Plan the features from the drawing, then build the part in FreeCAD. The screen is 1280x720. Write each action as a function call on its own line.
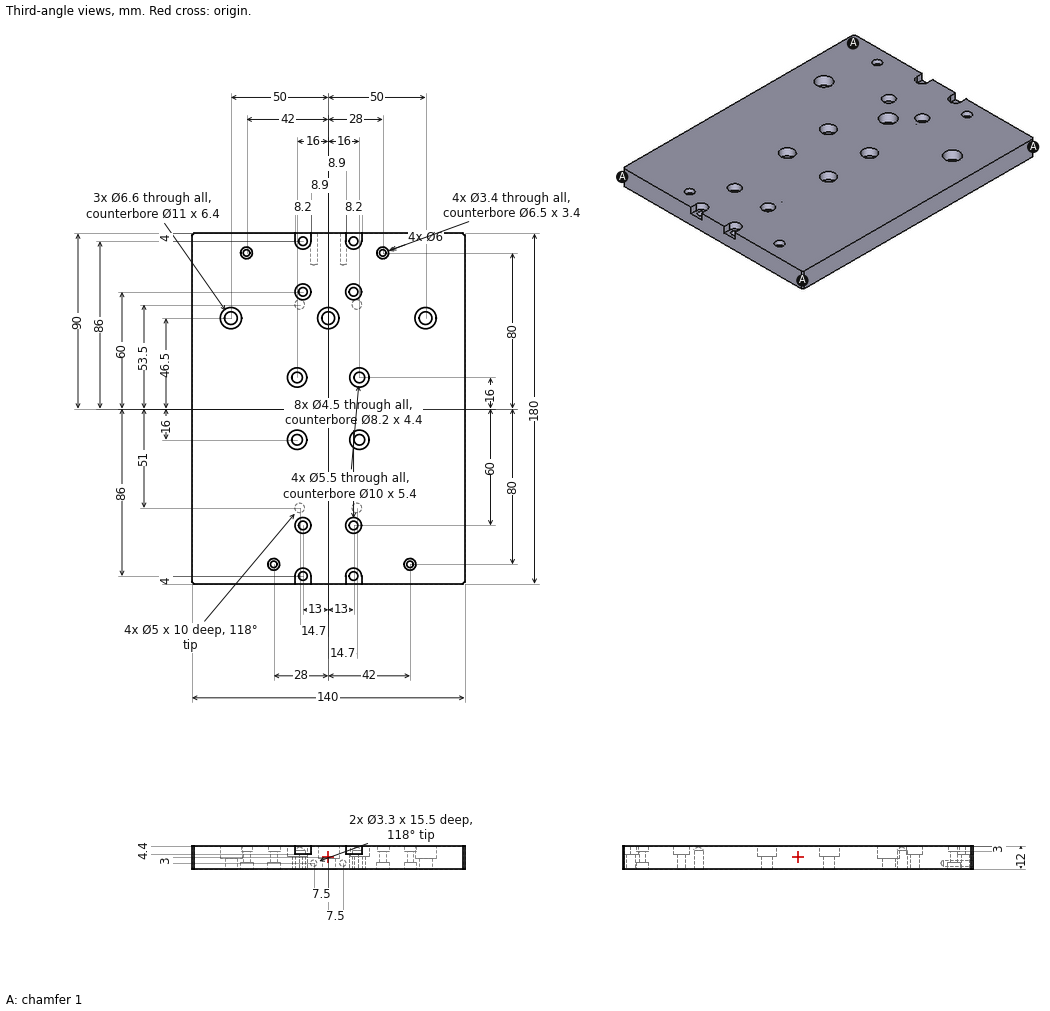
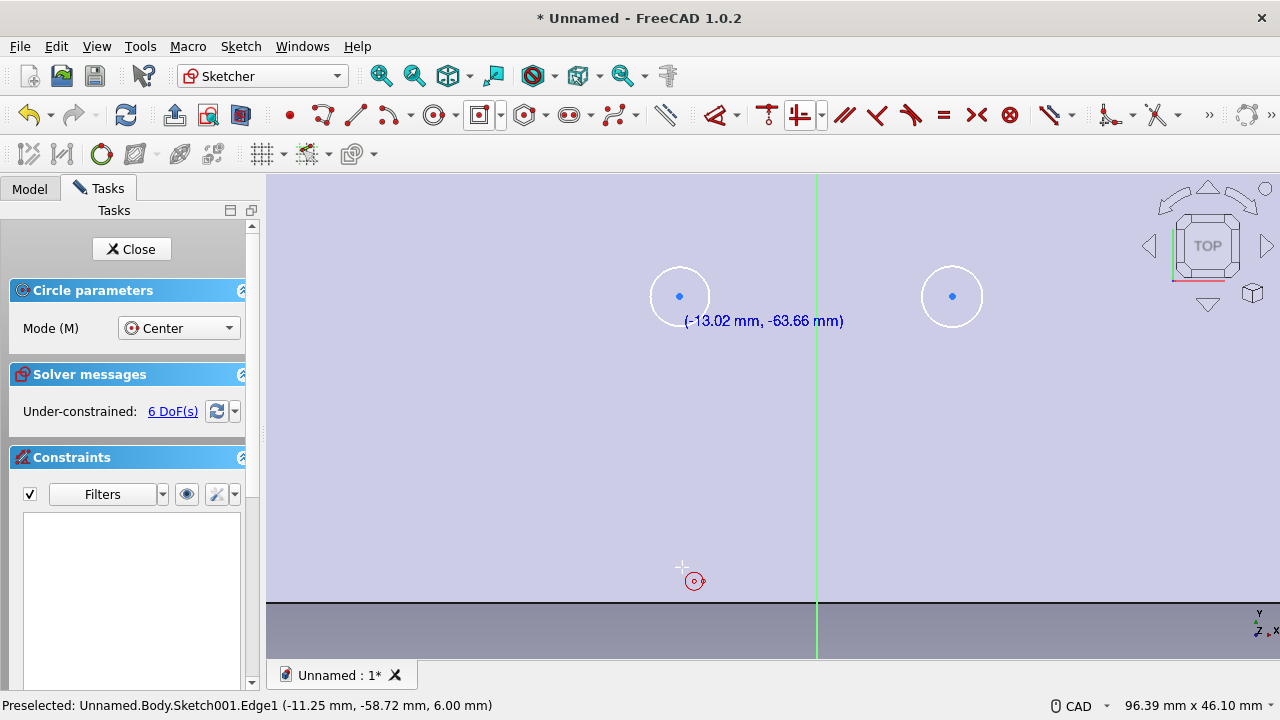
scroll(682, 567, down, 9)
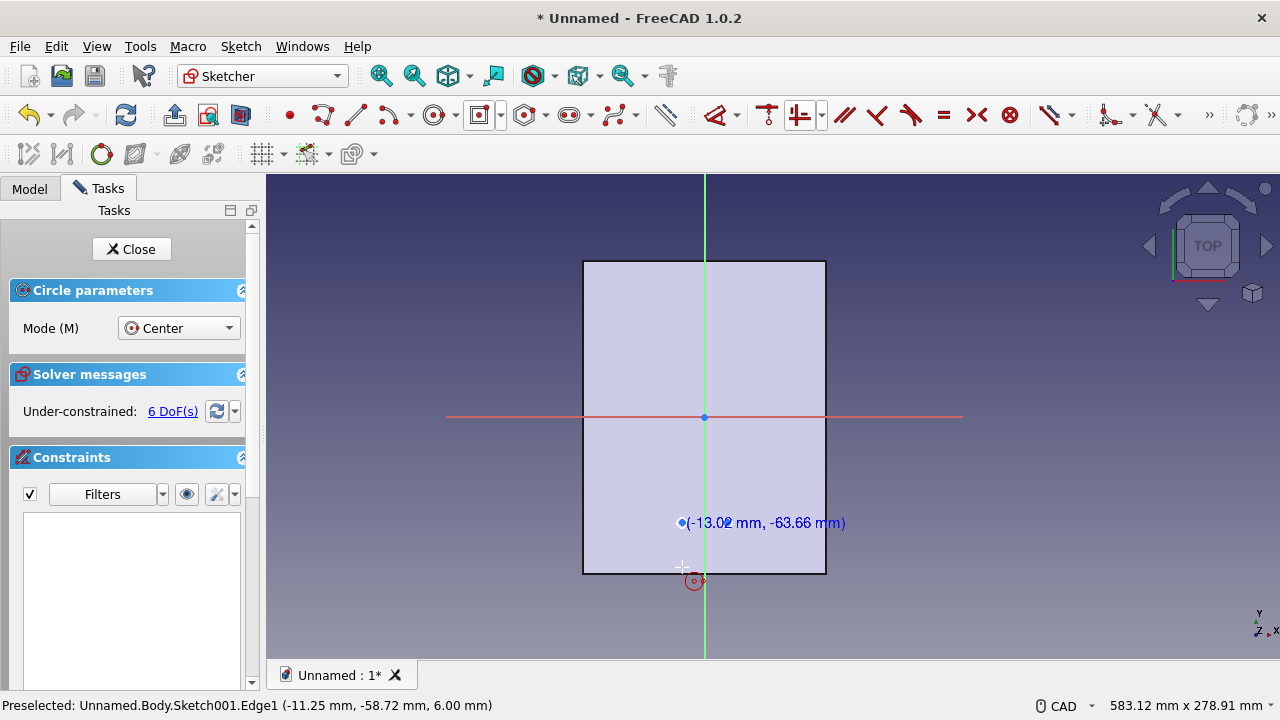
click(682, 567)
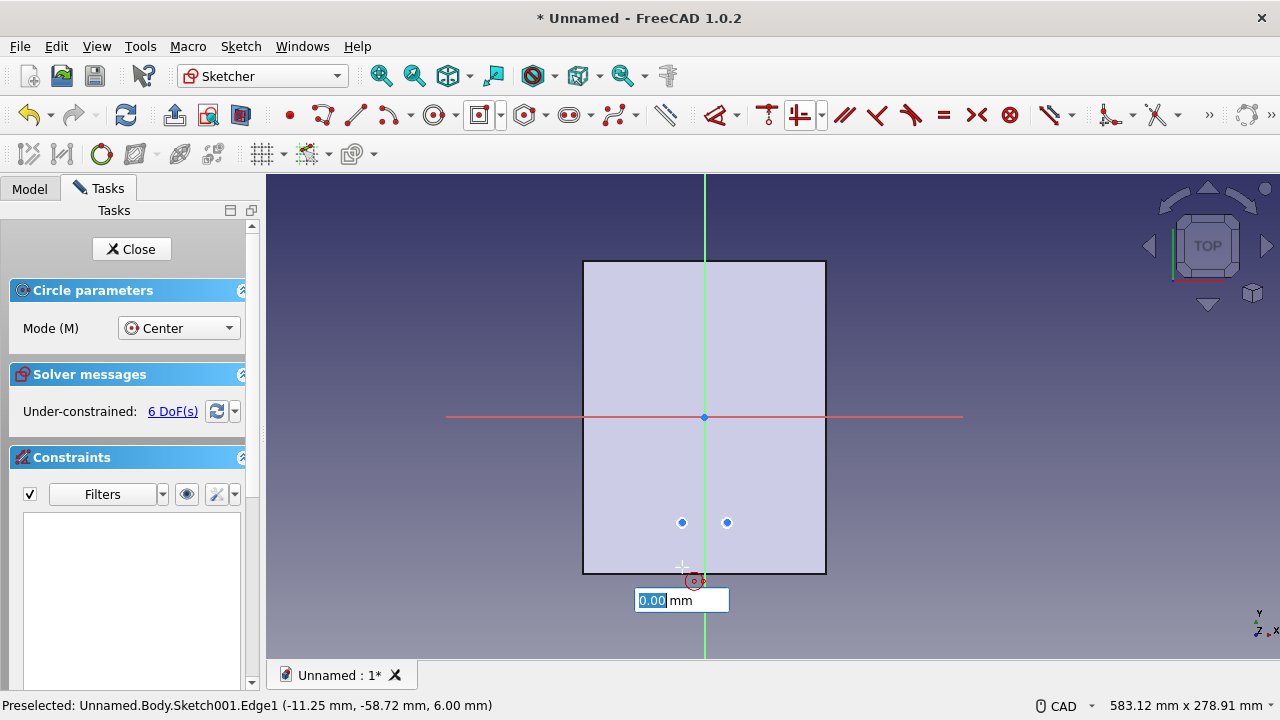
scroll(685, 564, up, 8)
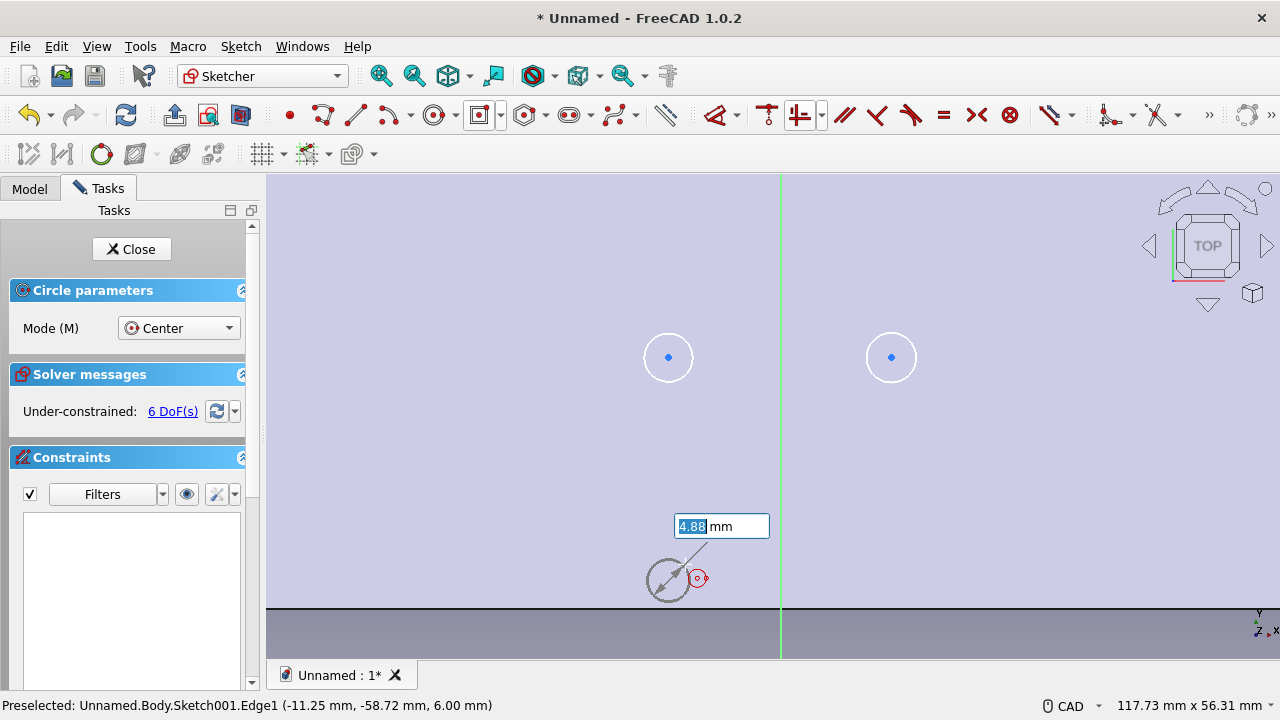
click(682, 561)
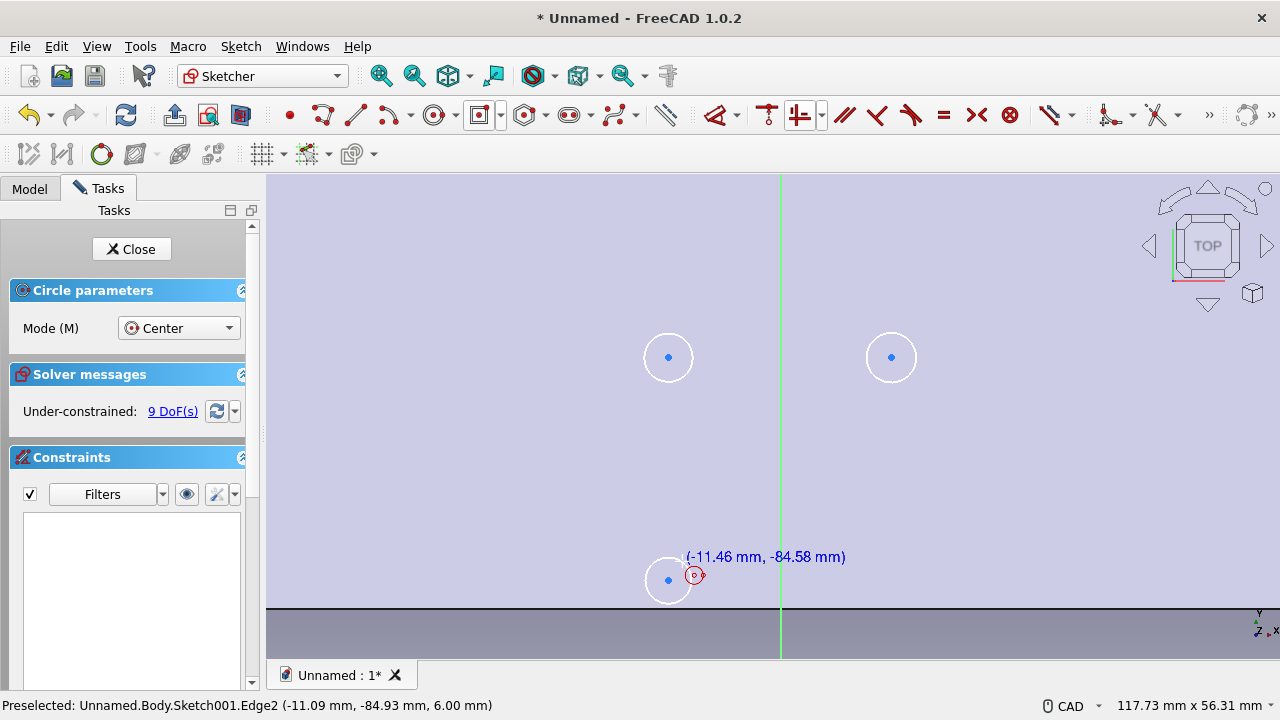
scroll(685, 564, down, 8)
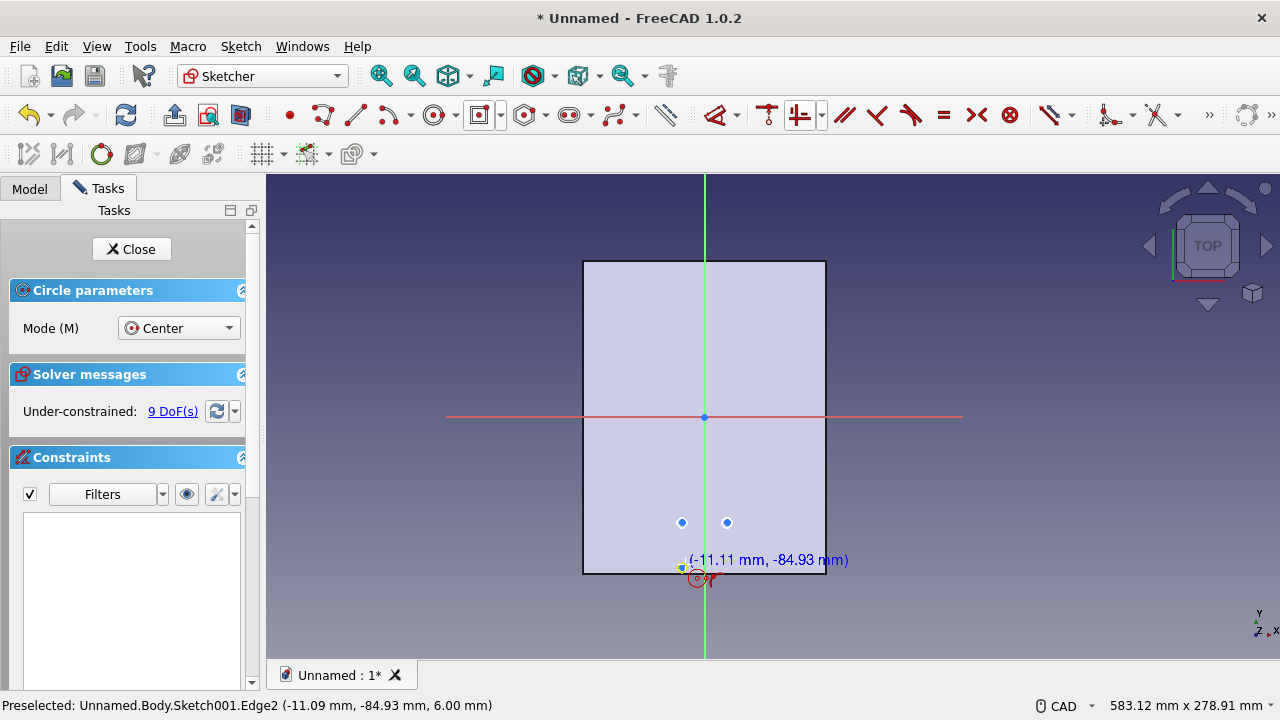
click(727, 567)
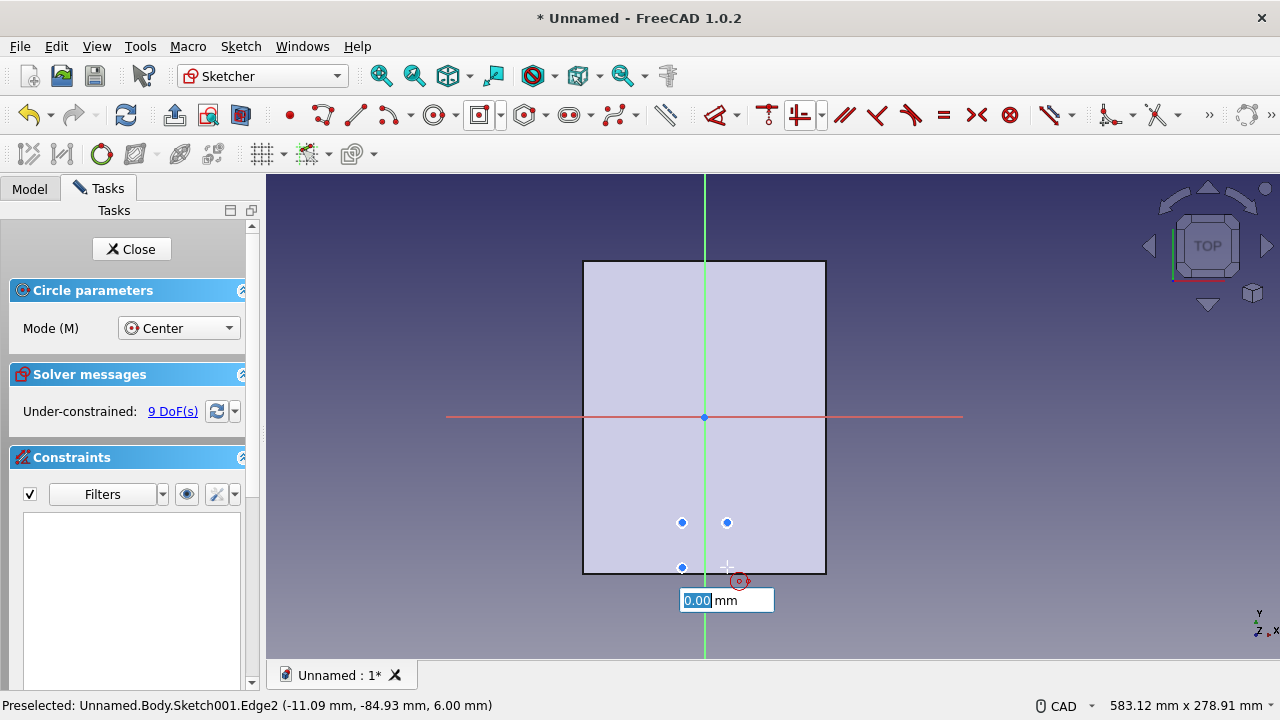
scroll(730, 564, up, 8)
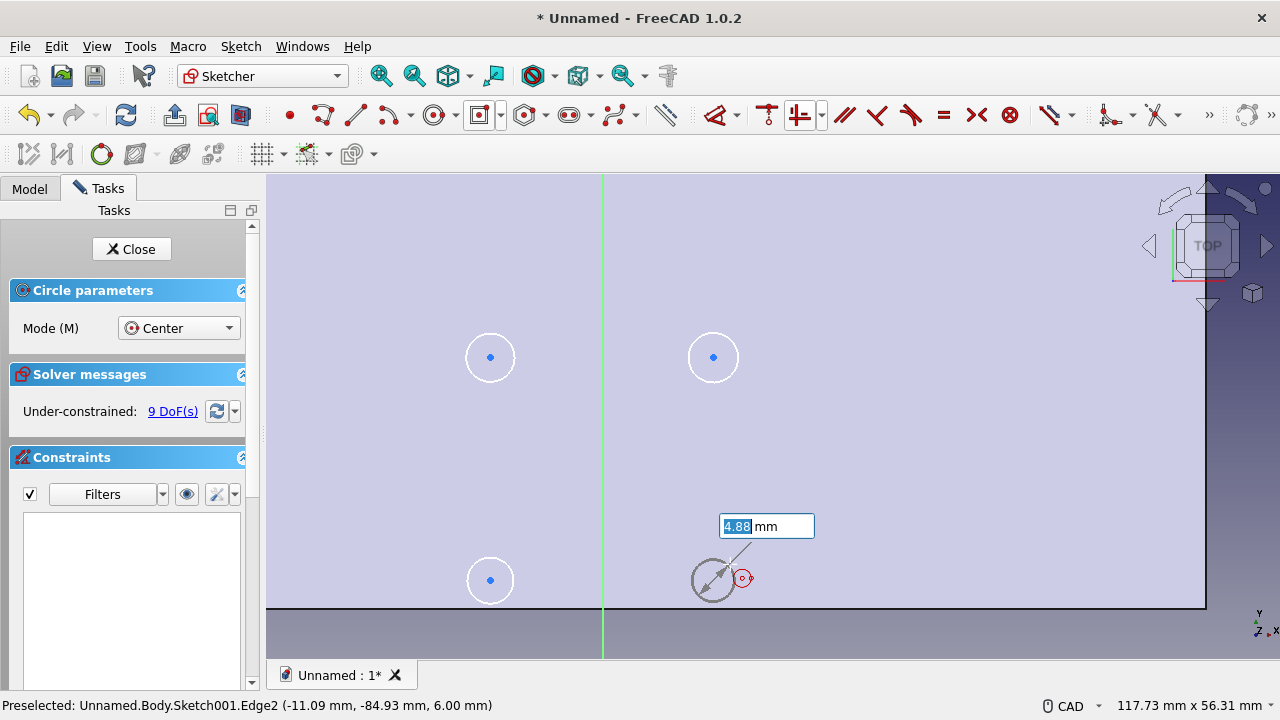
click(728, 561)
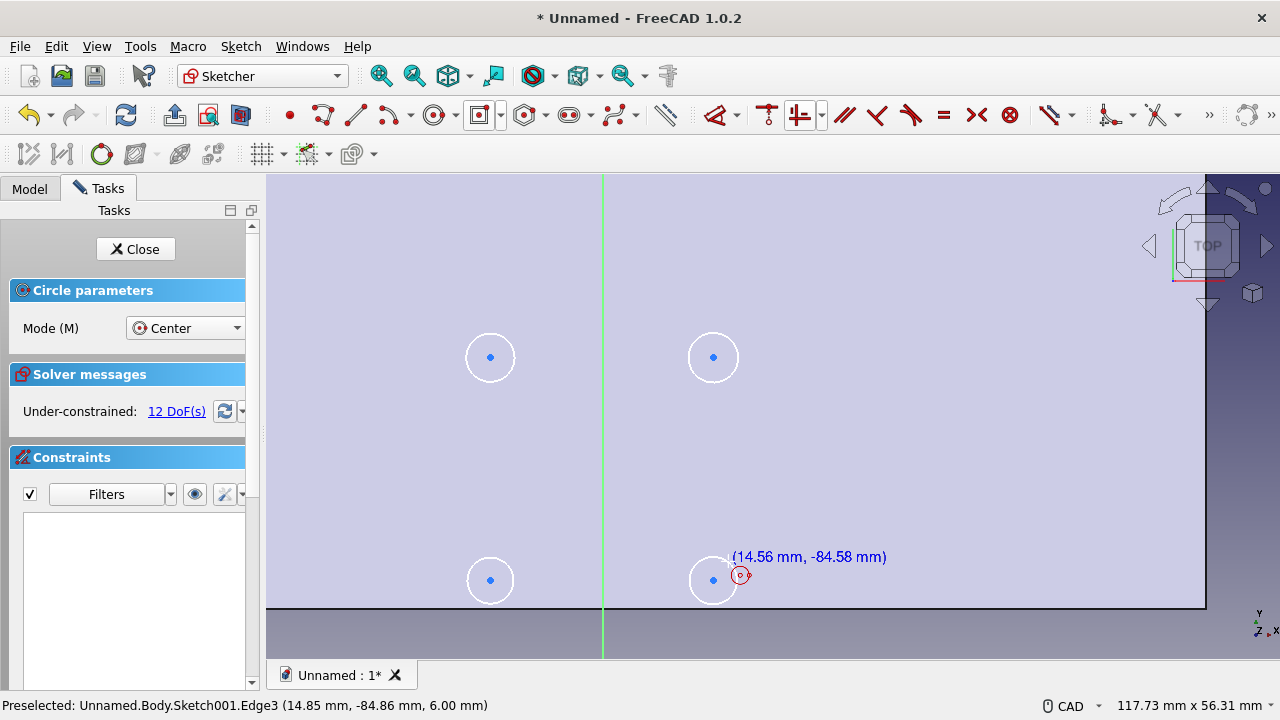
scroll(730, 564, down, 8)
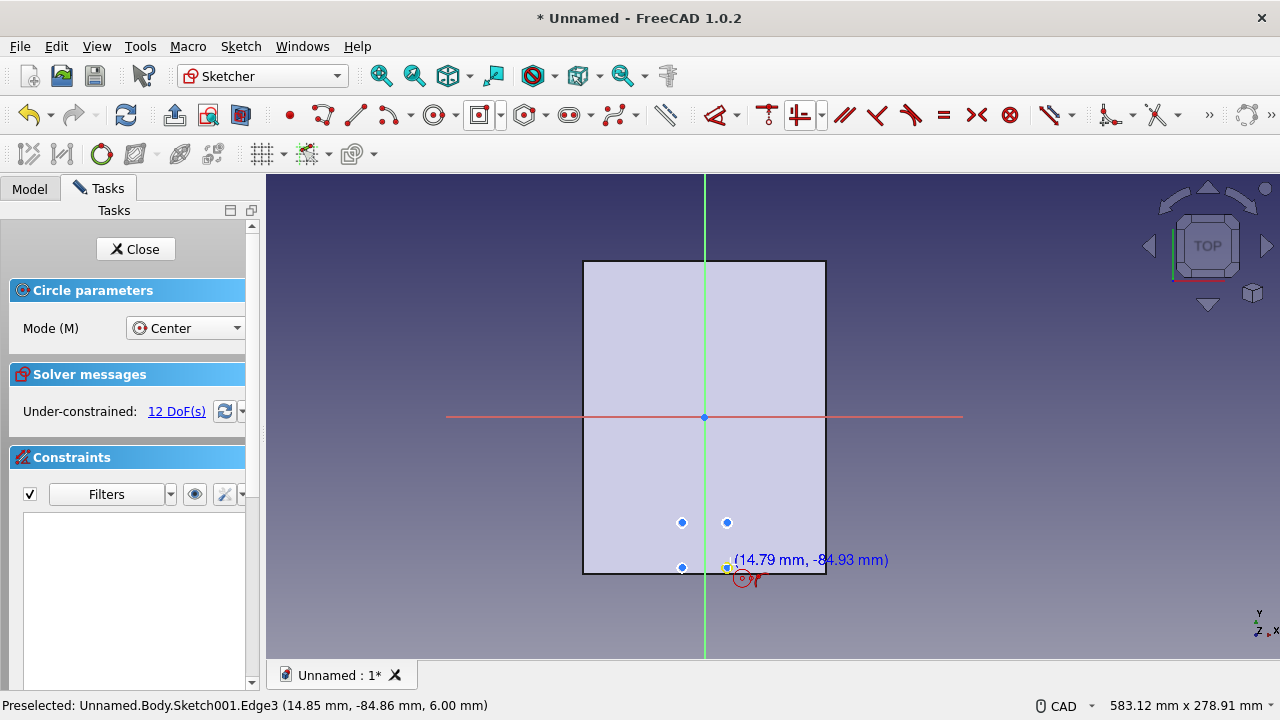
scroll(682, 268, up, 9)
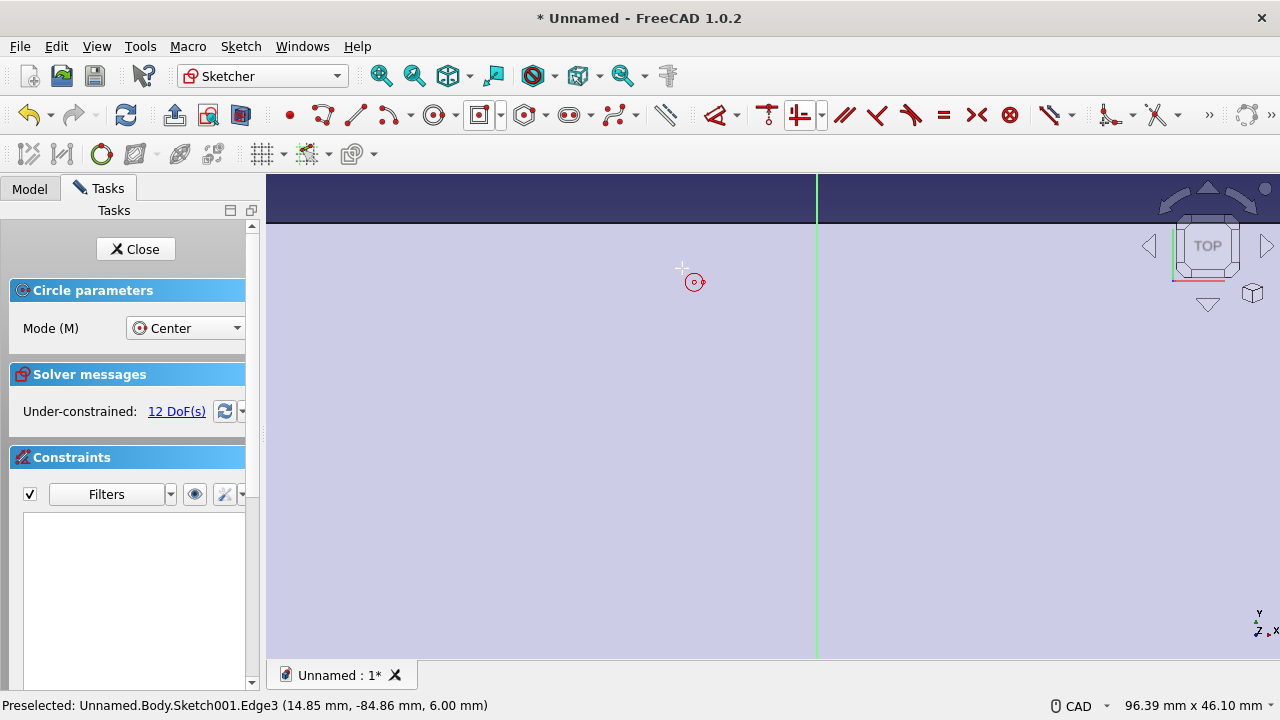
scroll(682, 267, down, 9)